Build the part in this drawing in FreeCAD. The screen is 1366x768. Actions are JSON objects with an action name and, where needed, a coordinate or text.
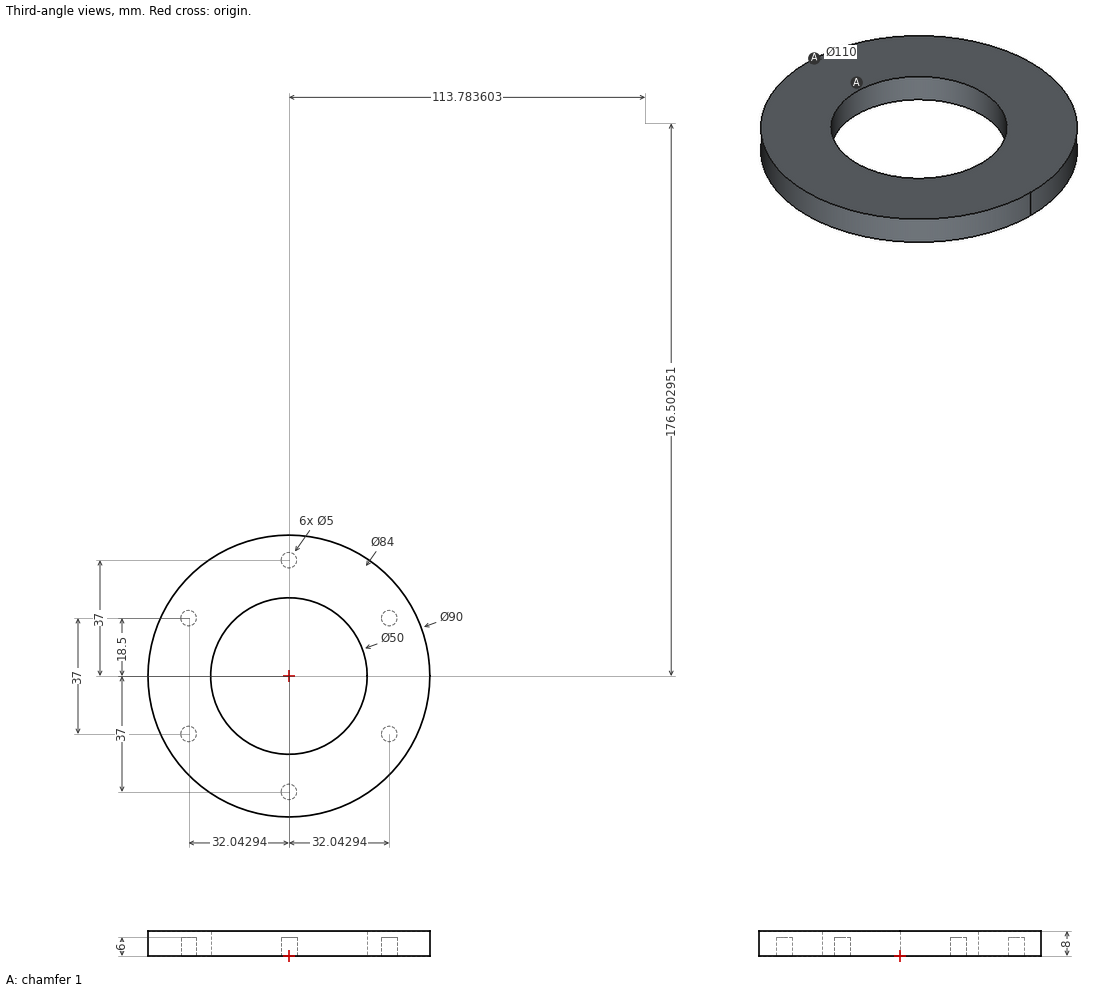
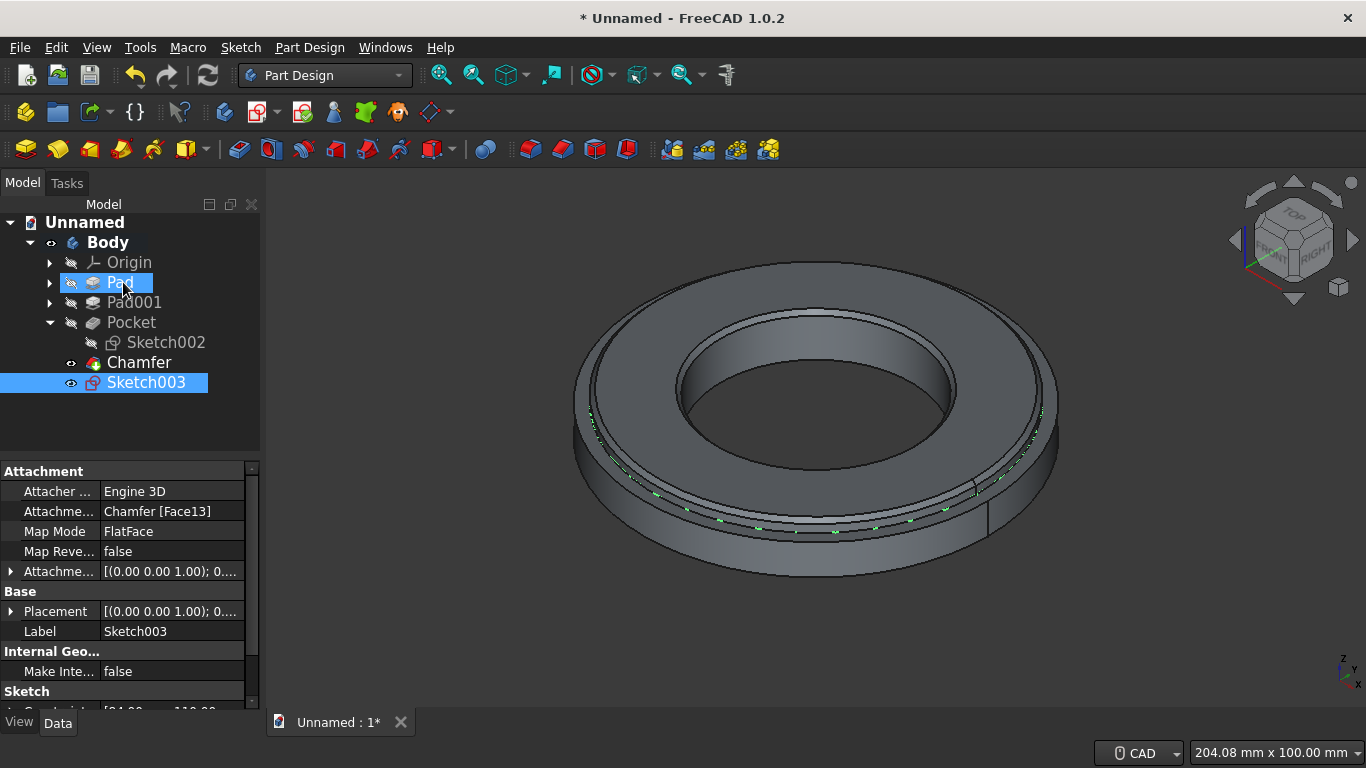
{"action": "left_click", "coordinate": [240, 150]}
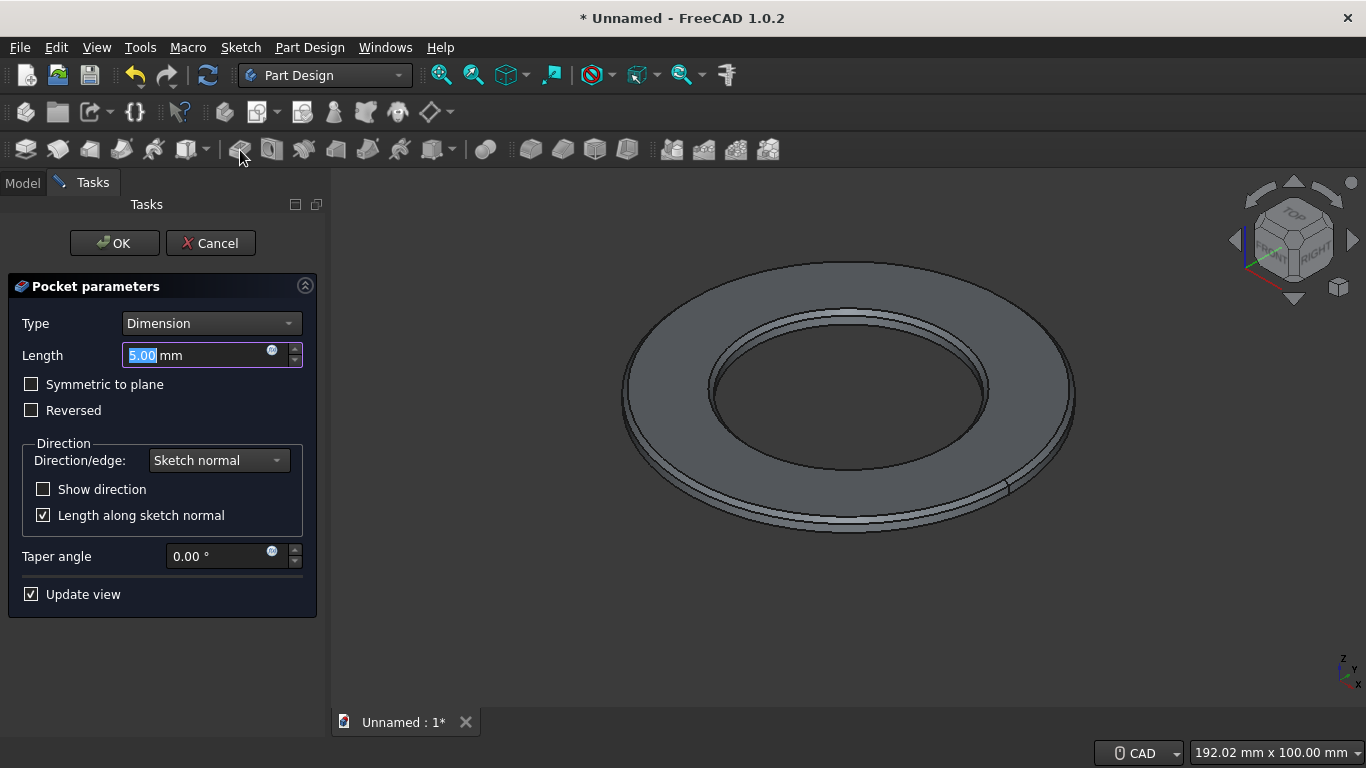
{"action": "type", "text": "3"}
{"action": "key", "text": "Tab"}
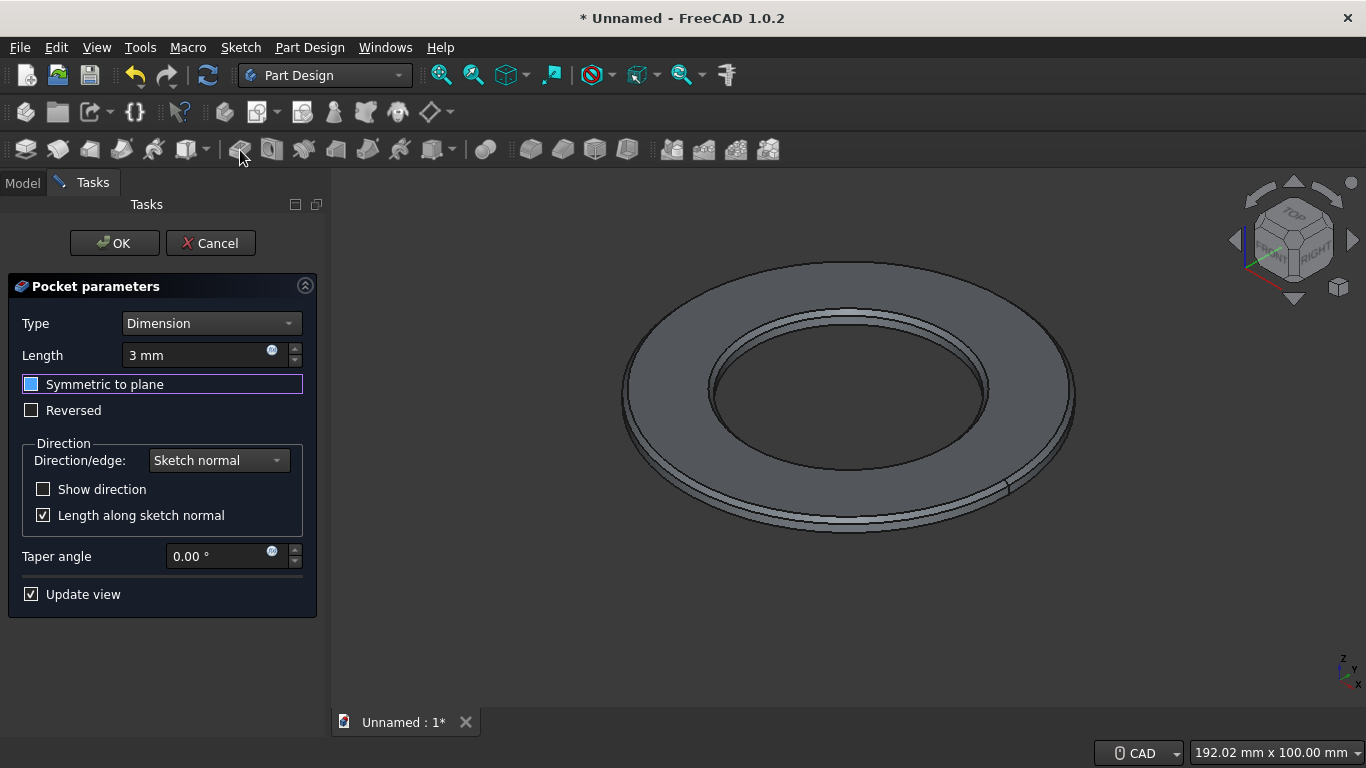
{"action": "left_click", "coordinate": [30, 410]}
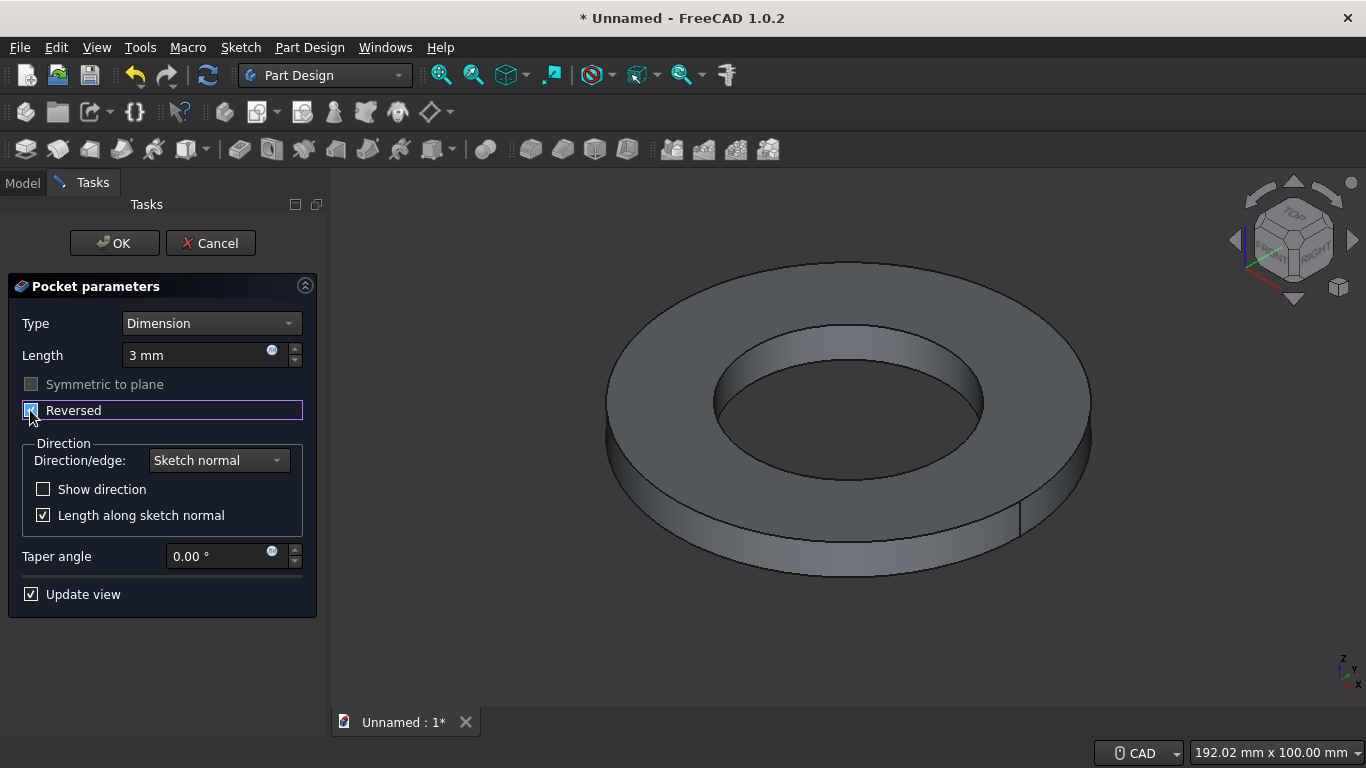
{"action": "left_click", "coordinate": [115, 243]}